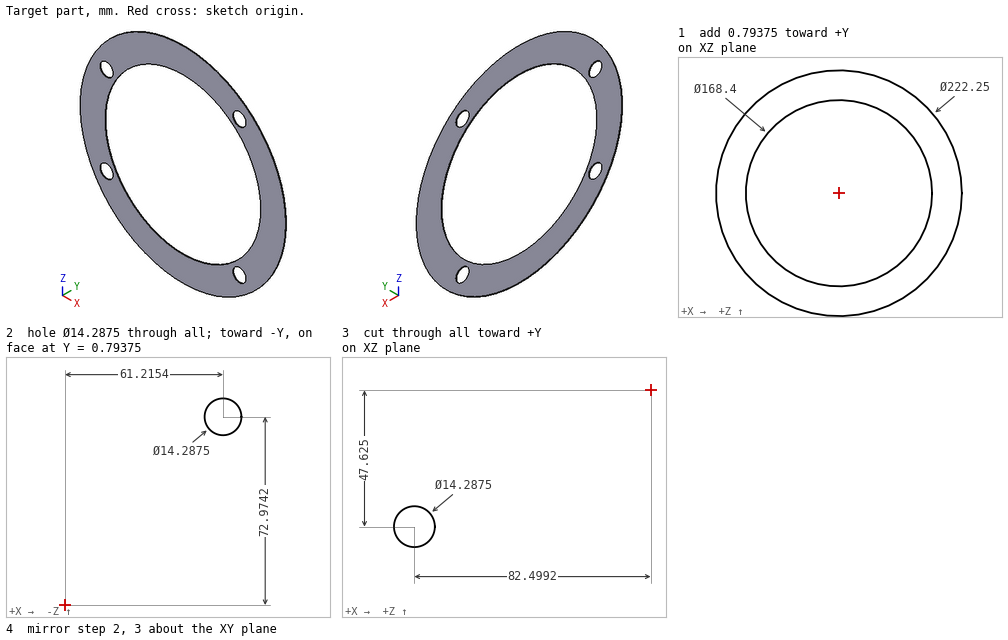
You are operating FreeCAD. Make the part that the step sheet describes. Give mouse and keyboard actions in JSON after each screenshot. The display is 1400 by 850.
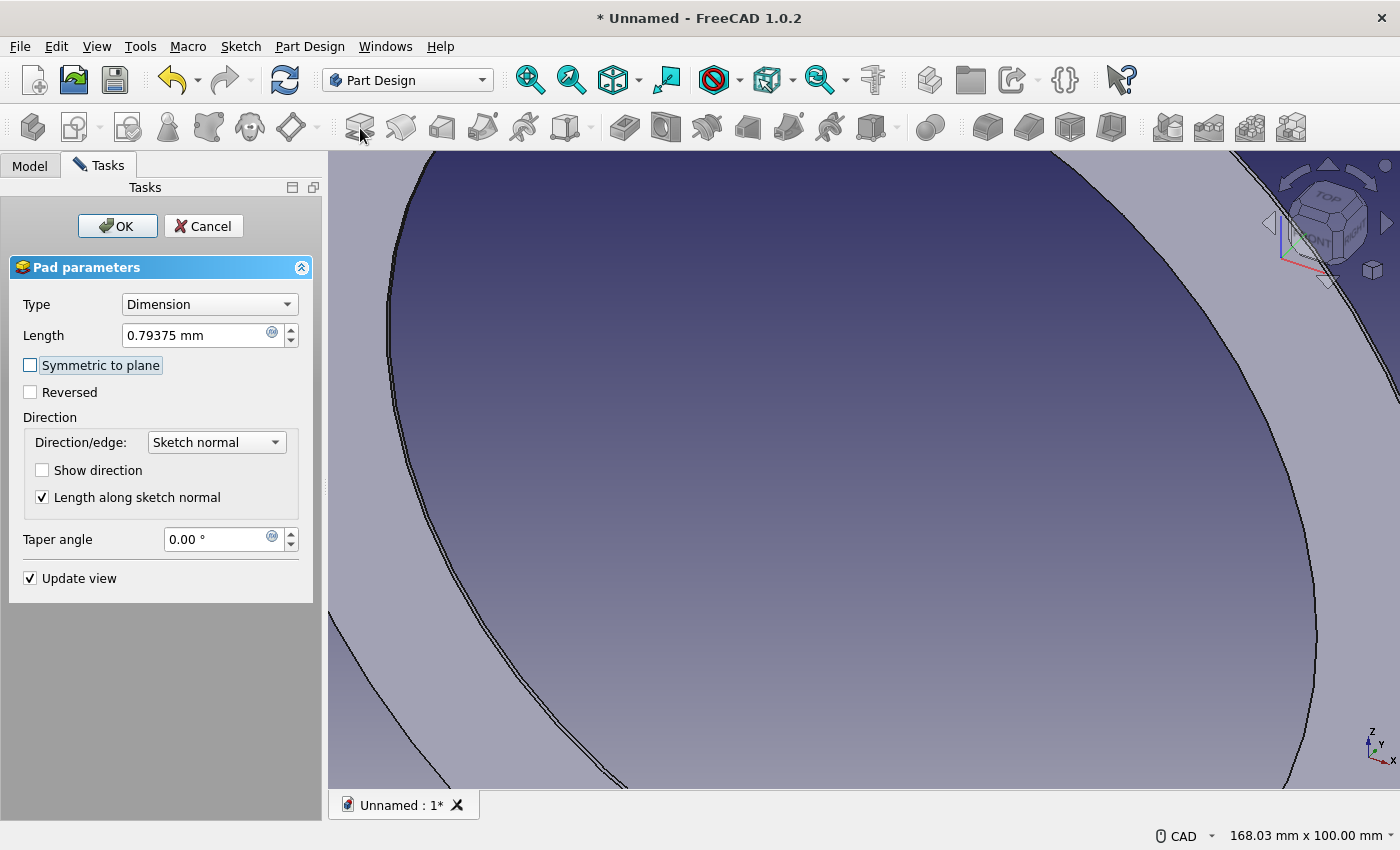
{"action": "left_click", "coordinate": [31, 392]}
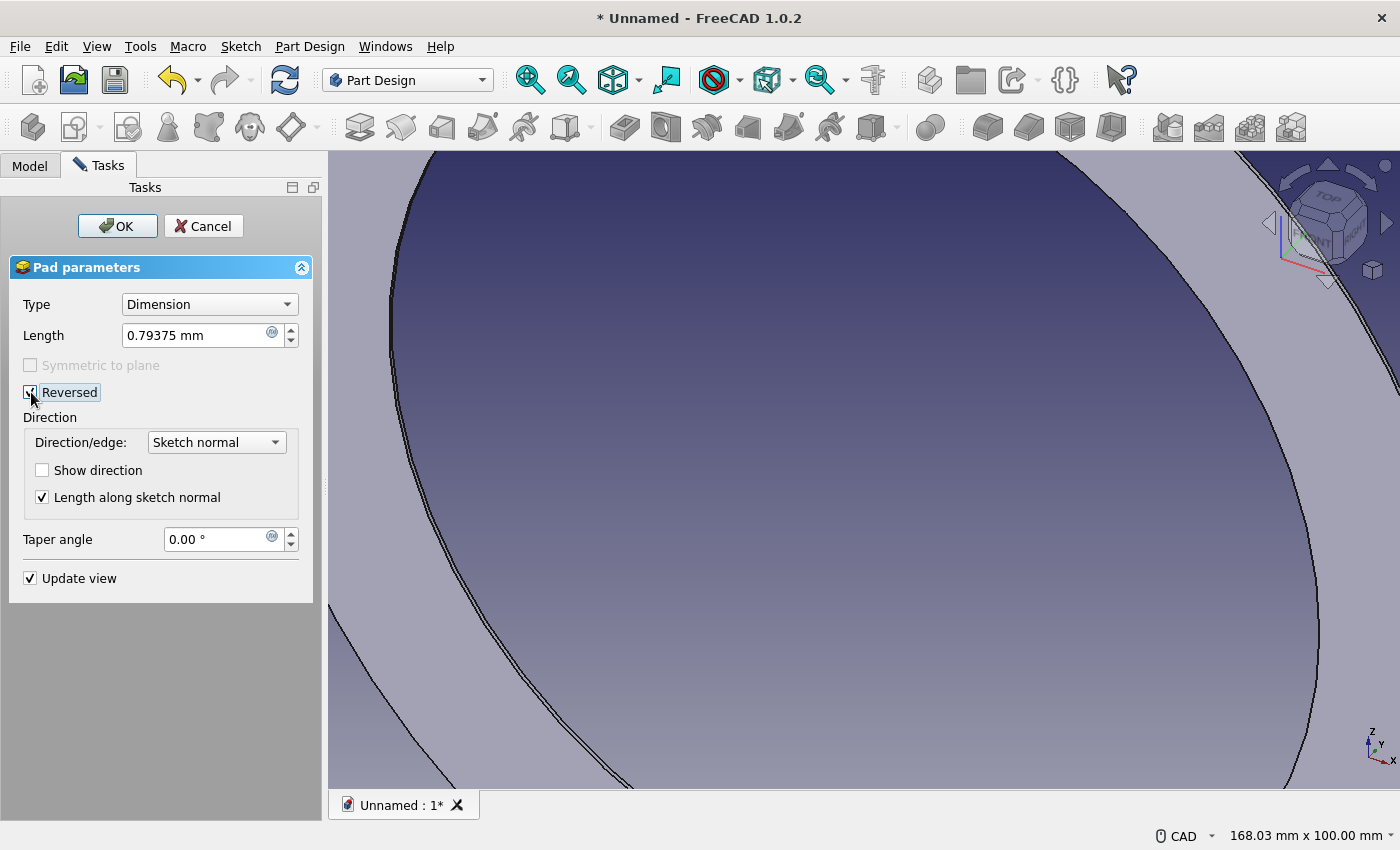
{"action": "left_click", "coordinate": [118, 226]}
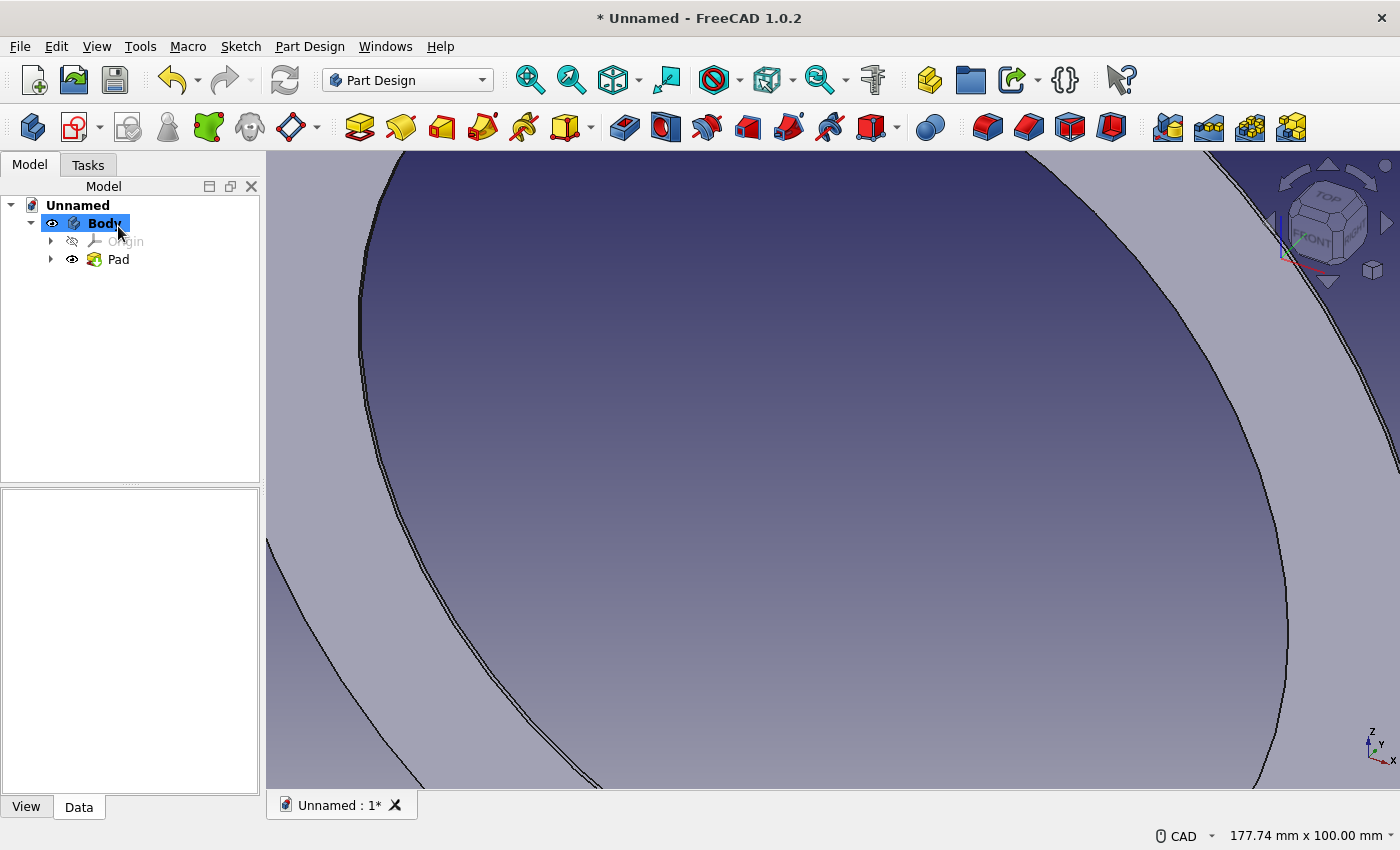
{"action": "left_click", "coordinate": [531, 80]}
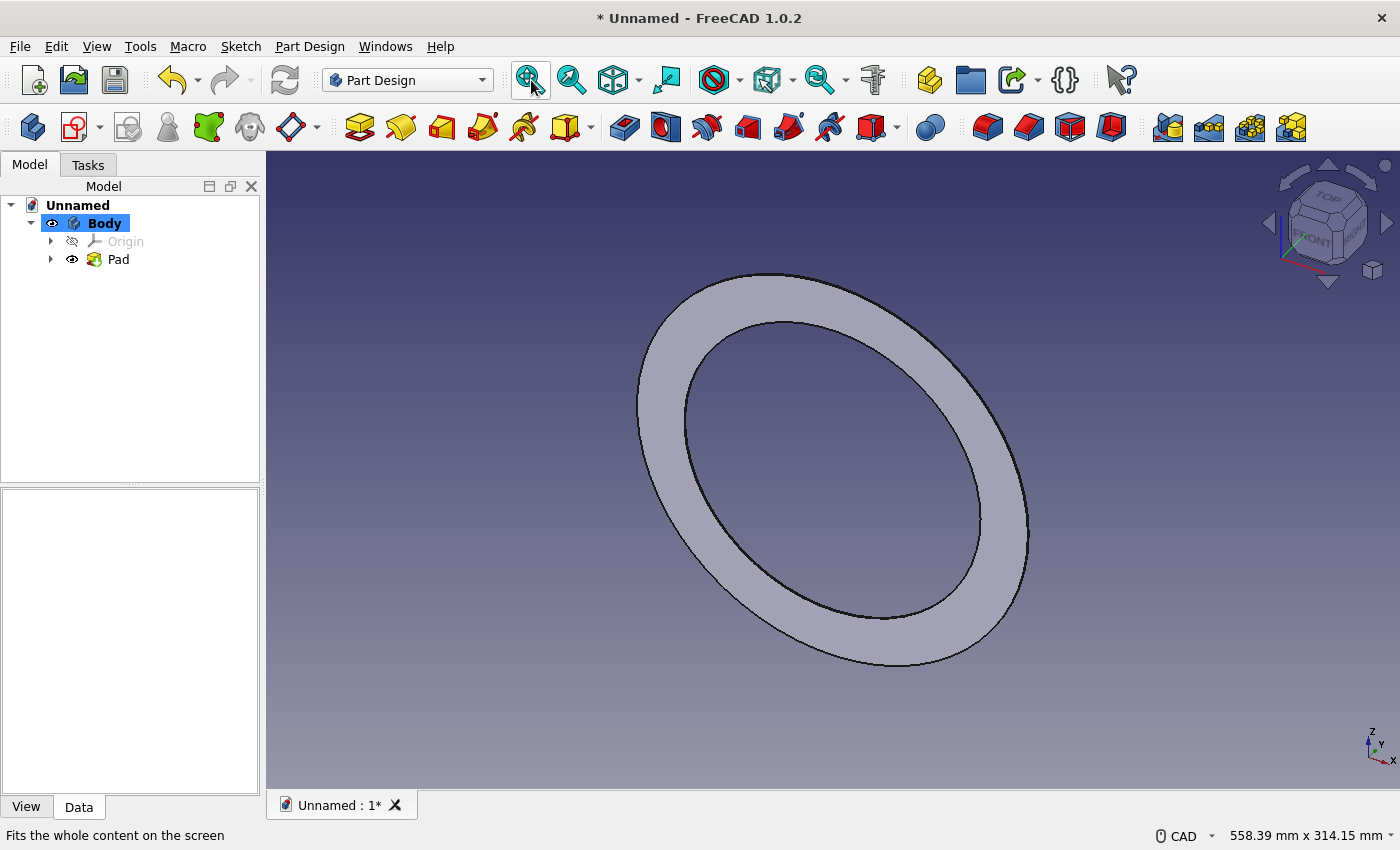
{"action": "key", "text": "4"}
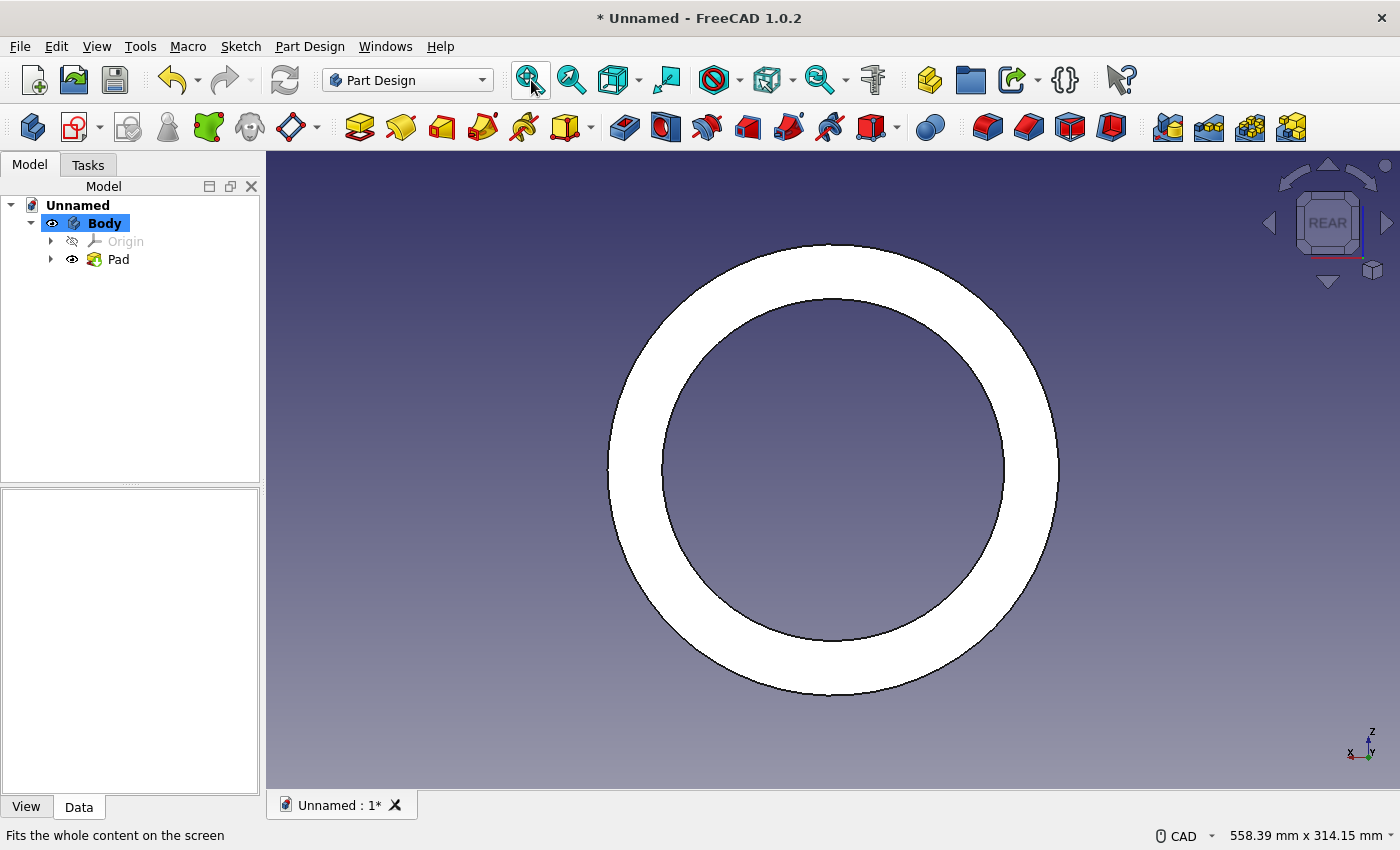
{"action": "left_click", "coordinate": [640, 469]}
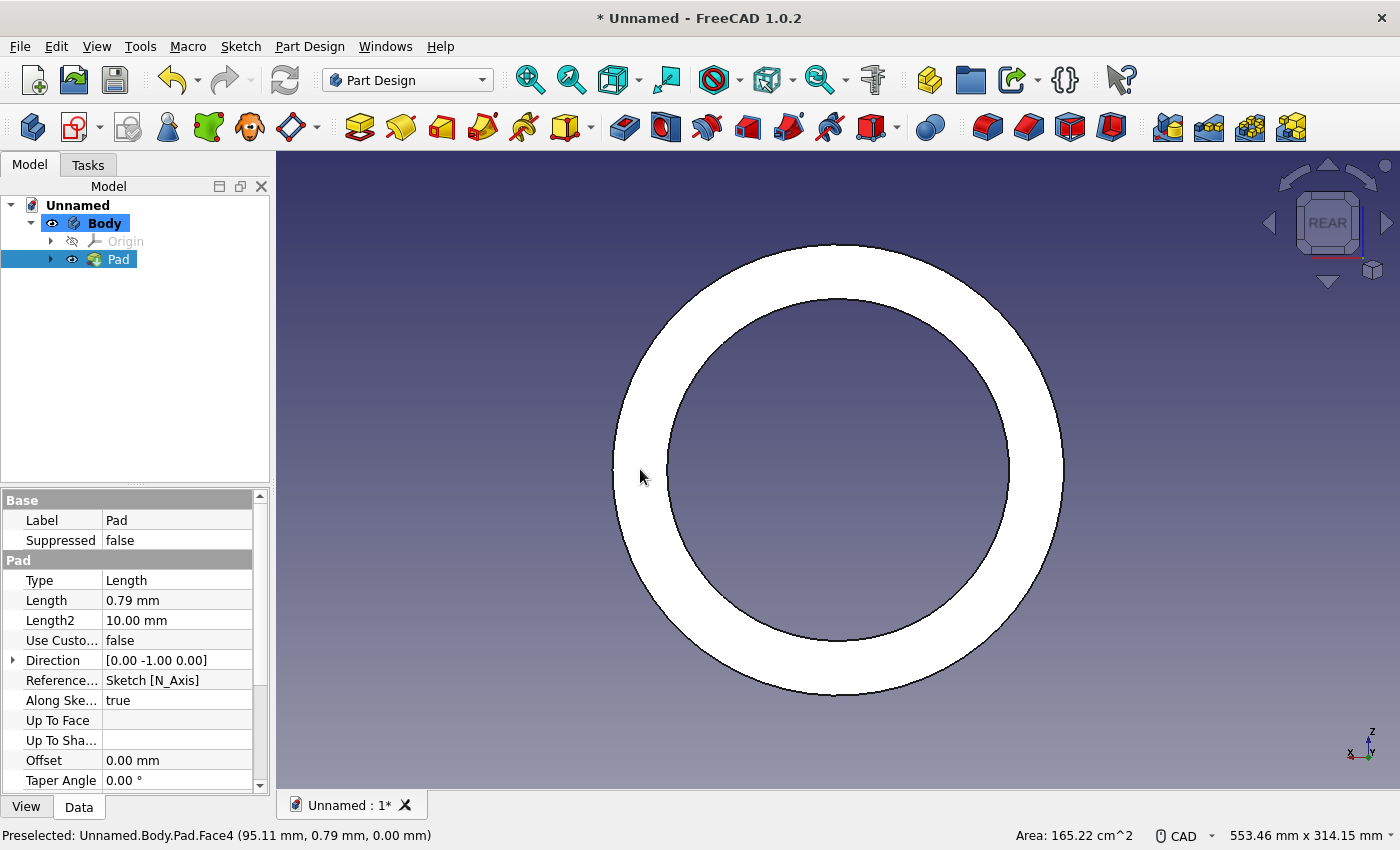
{"action": "left_click", "coordinate": [74, 128]}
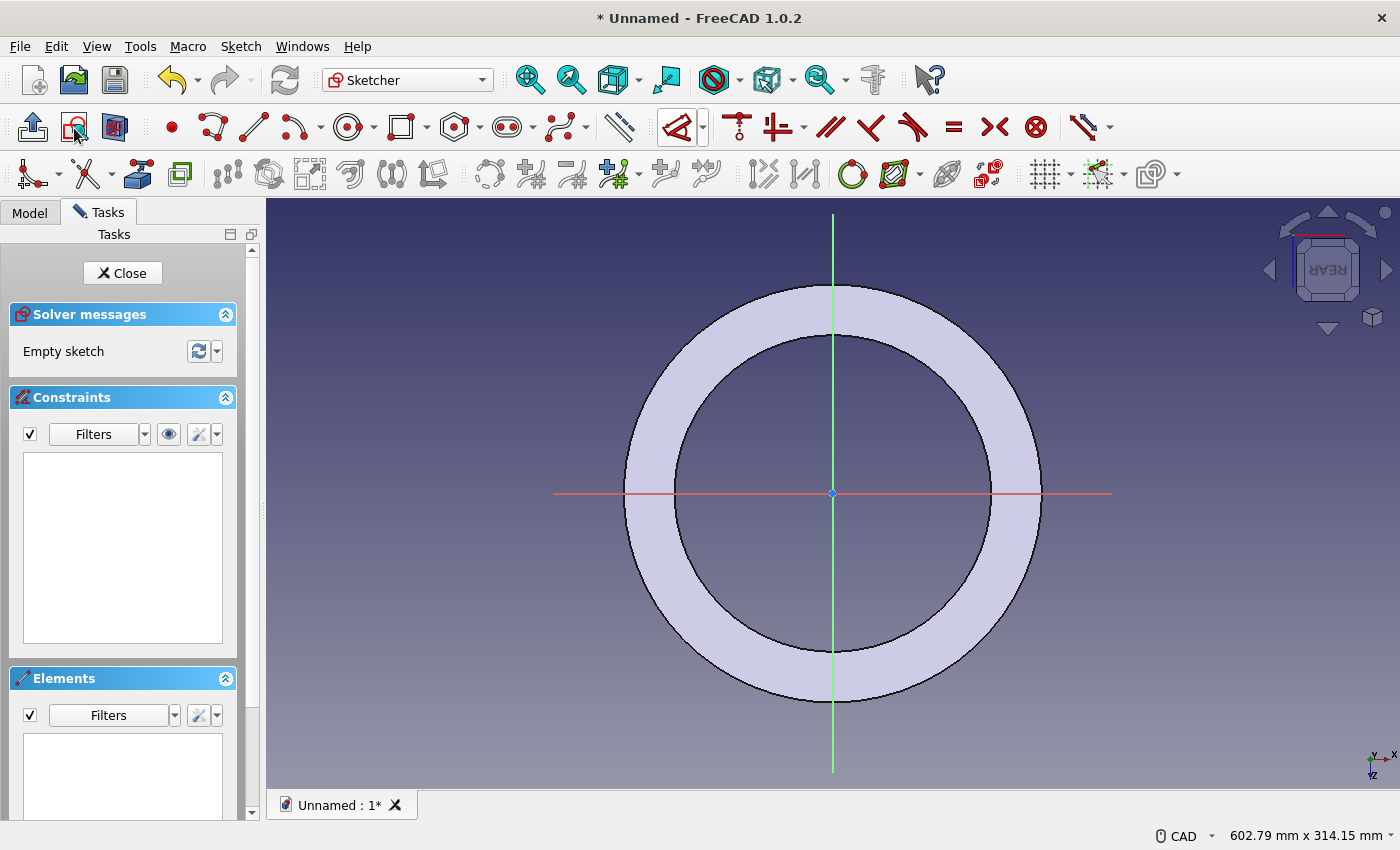
{"action": "scroll", "coordinate": [963, 345], "scroll_direction": "up", "scroll_amount": 13}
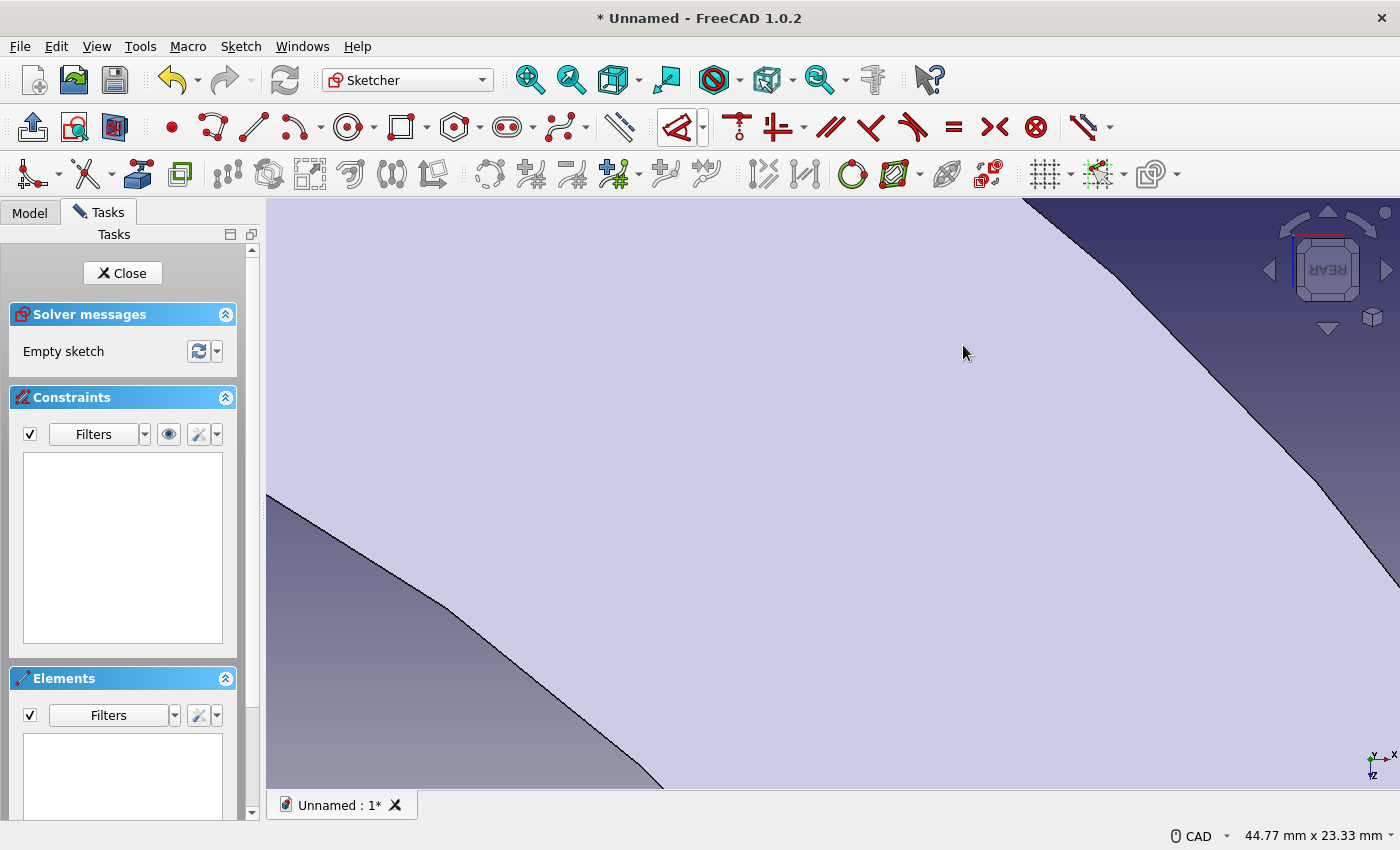
{"action": "left_click", "coordinate": [348, 128]}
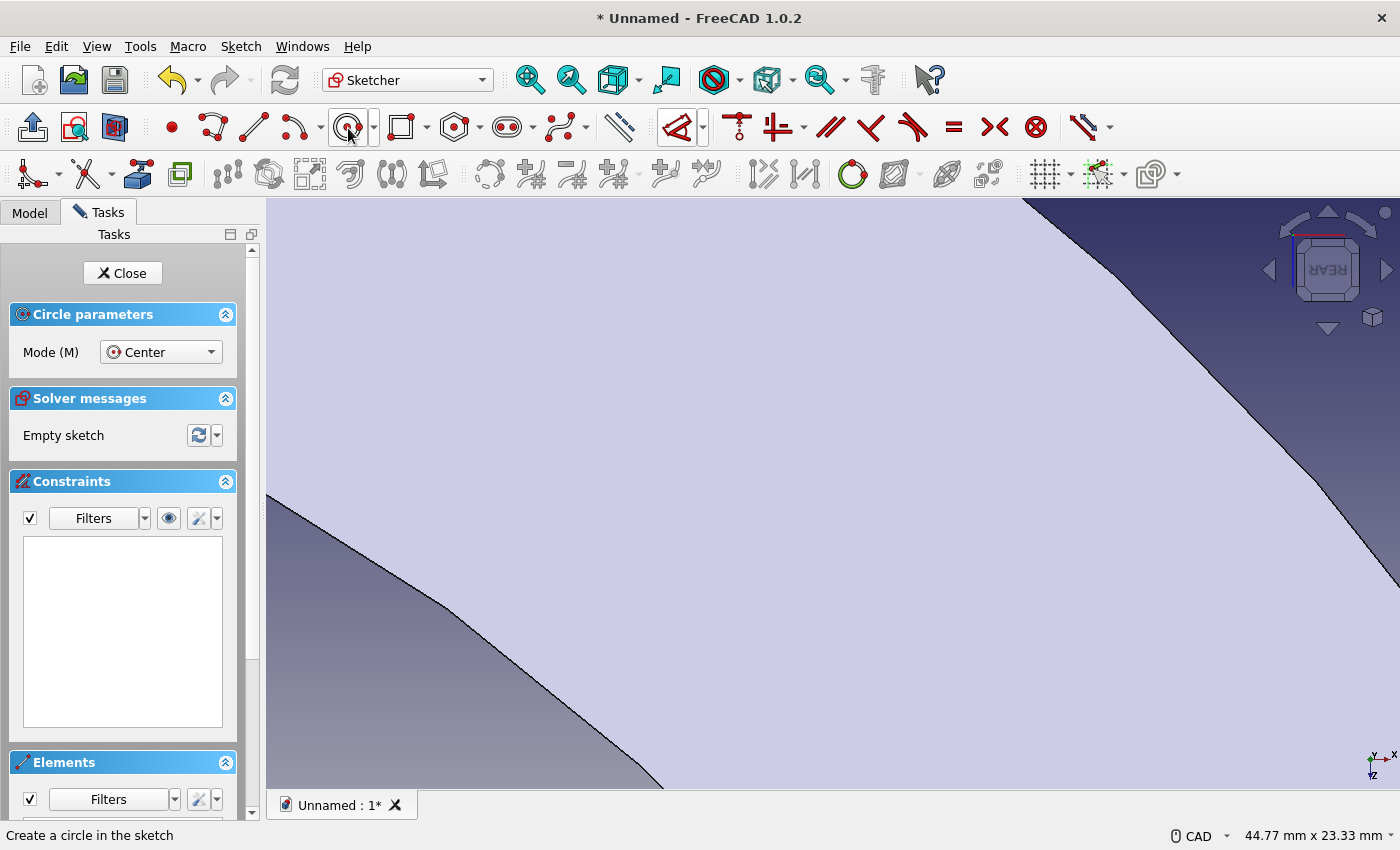
{"action": "left_click", "coordinate": [754, 493]}
{"action": "left_click", "coordinate": [882, 365]}
{"action": "key", "text": "Escape"}